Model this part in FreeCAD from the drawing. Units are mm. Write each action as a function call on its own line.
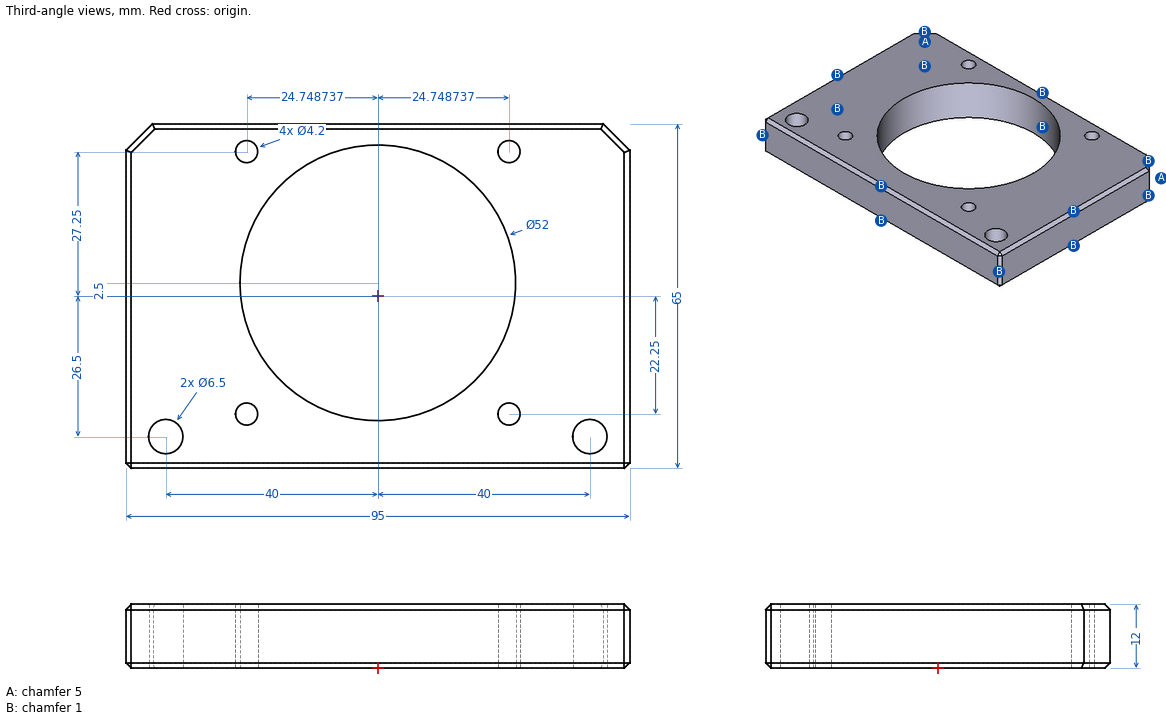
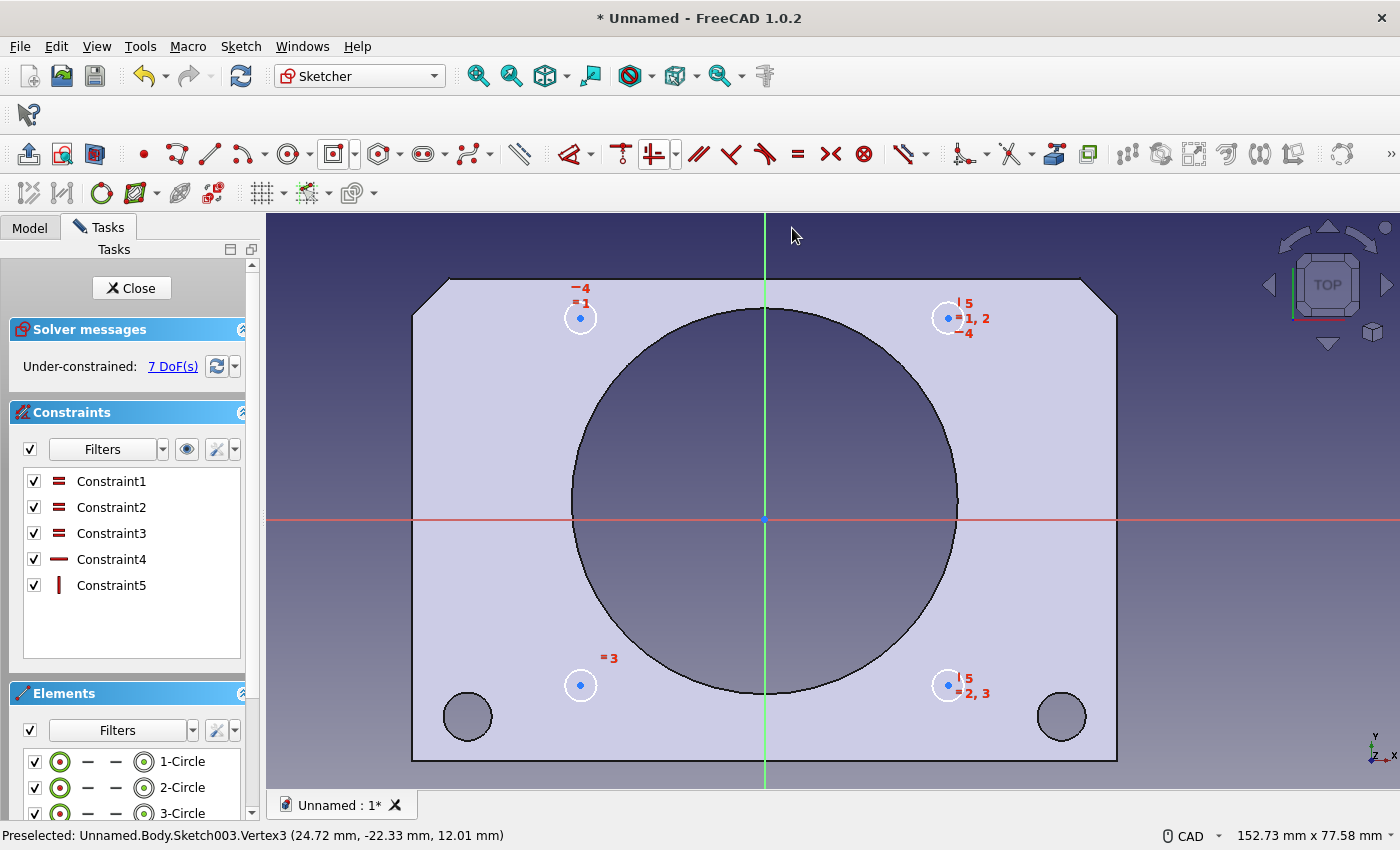
click(581, 318)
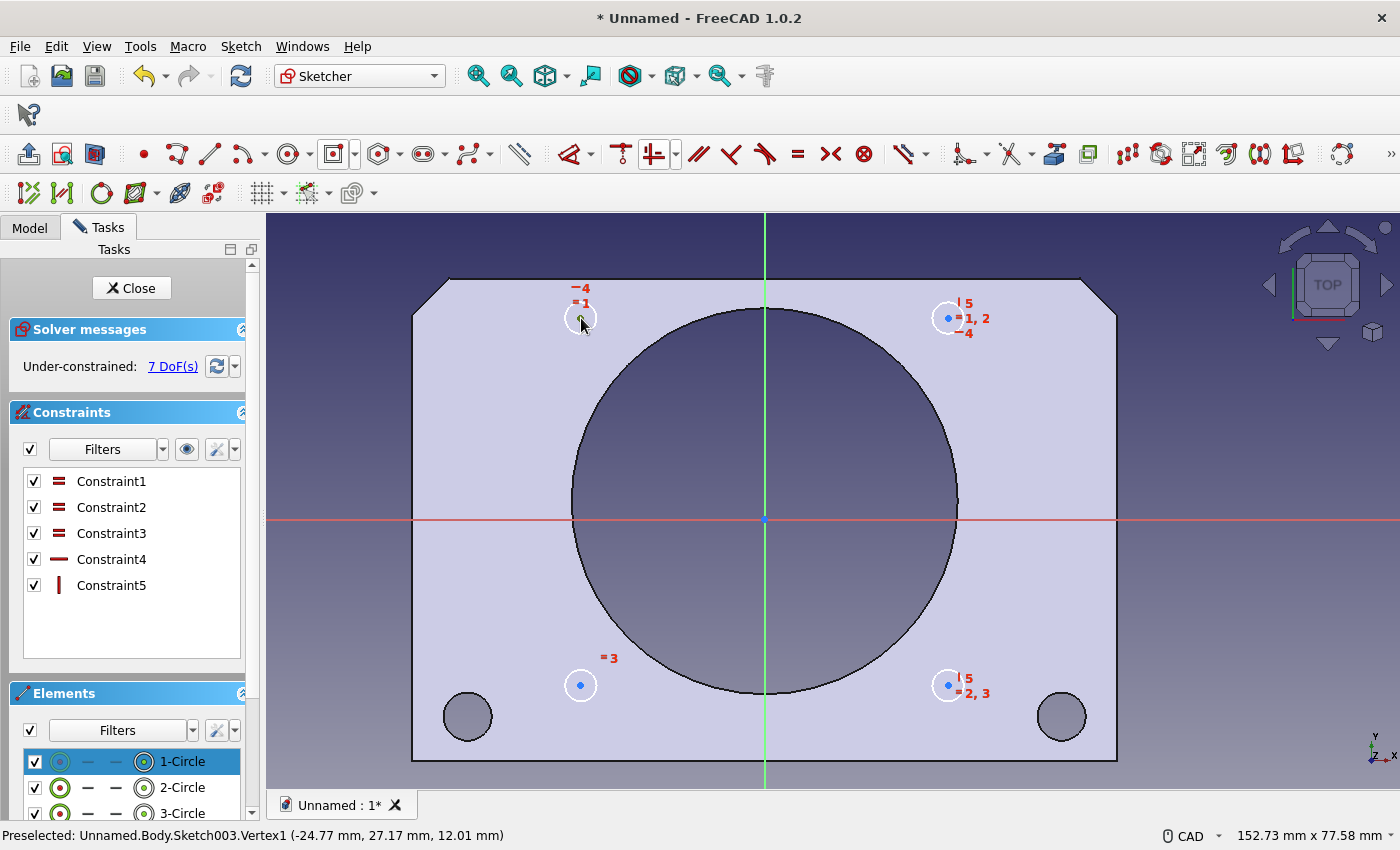
click(581, 686)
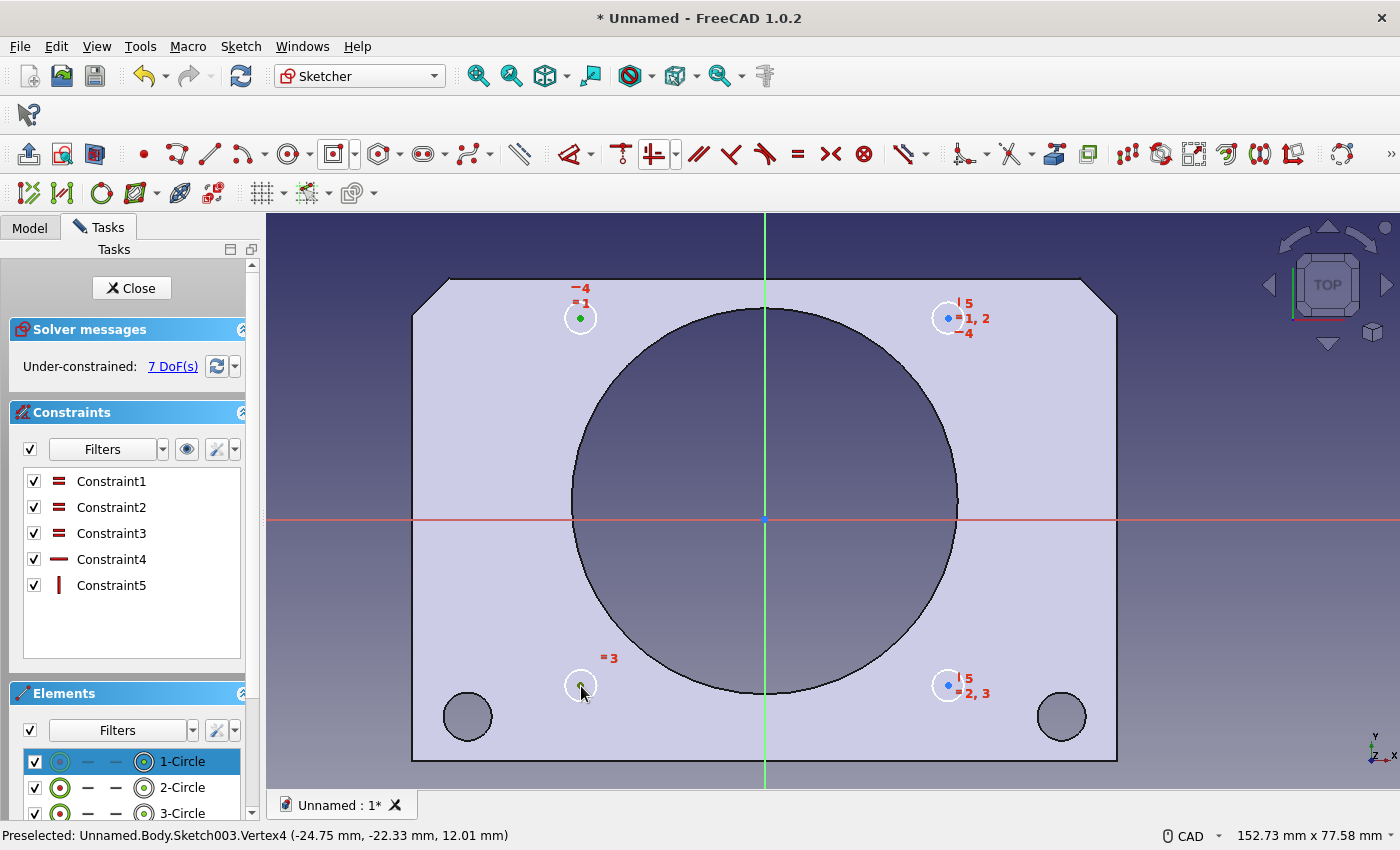
click(676, 154)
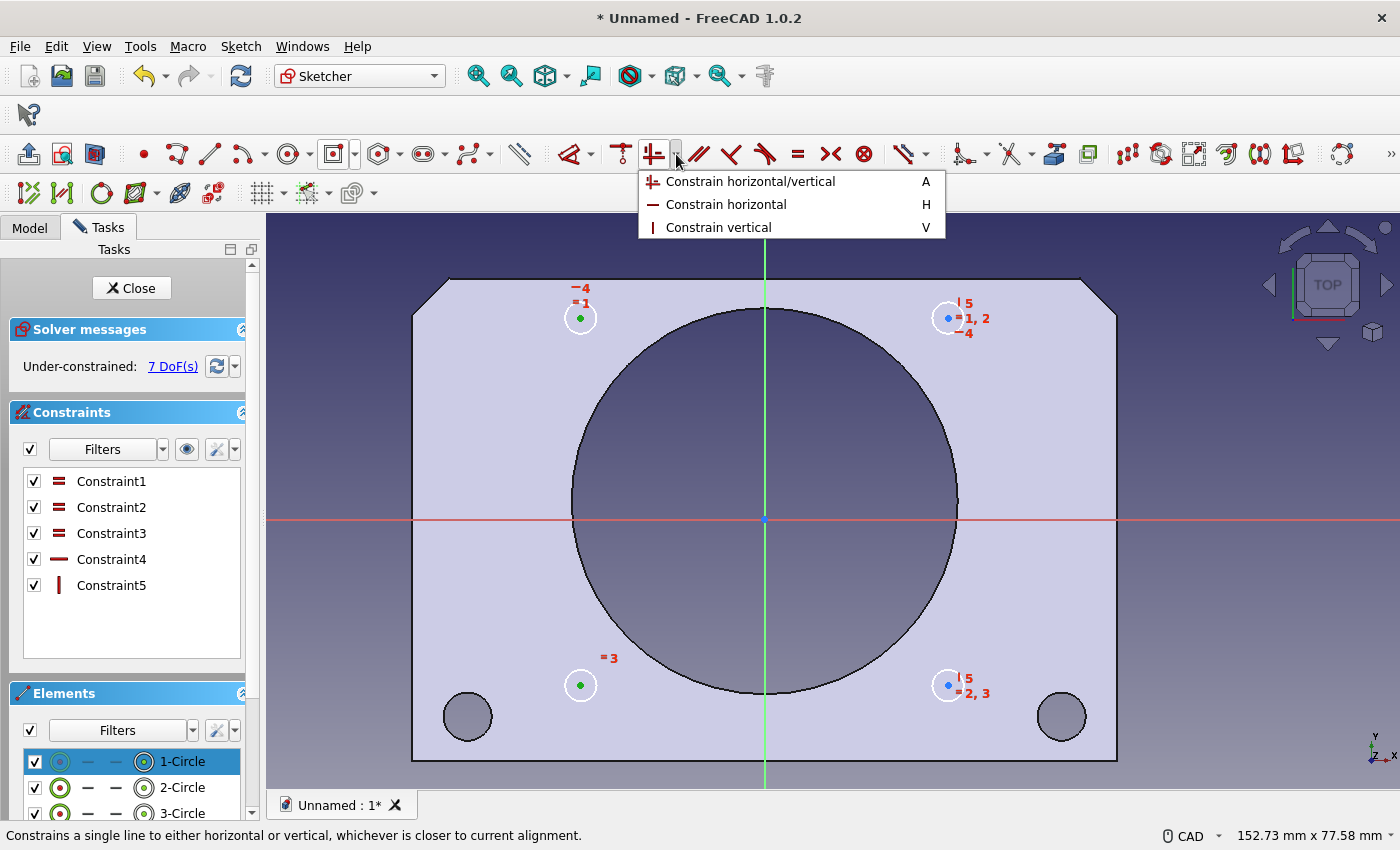
click(792, 228)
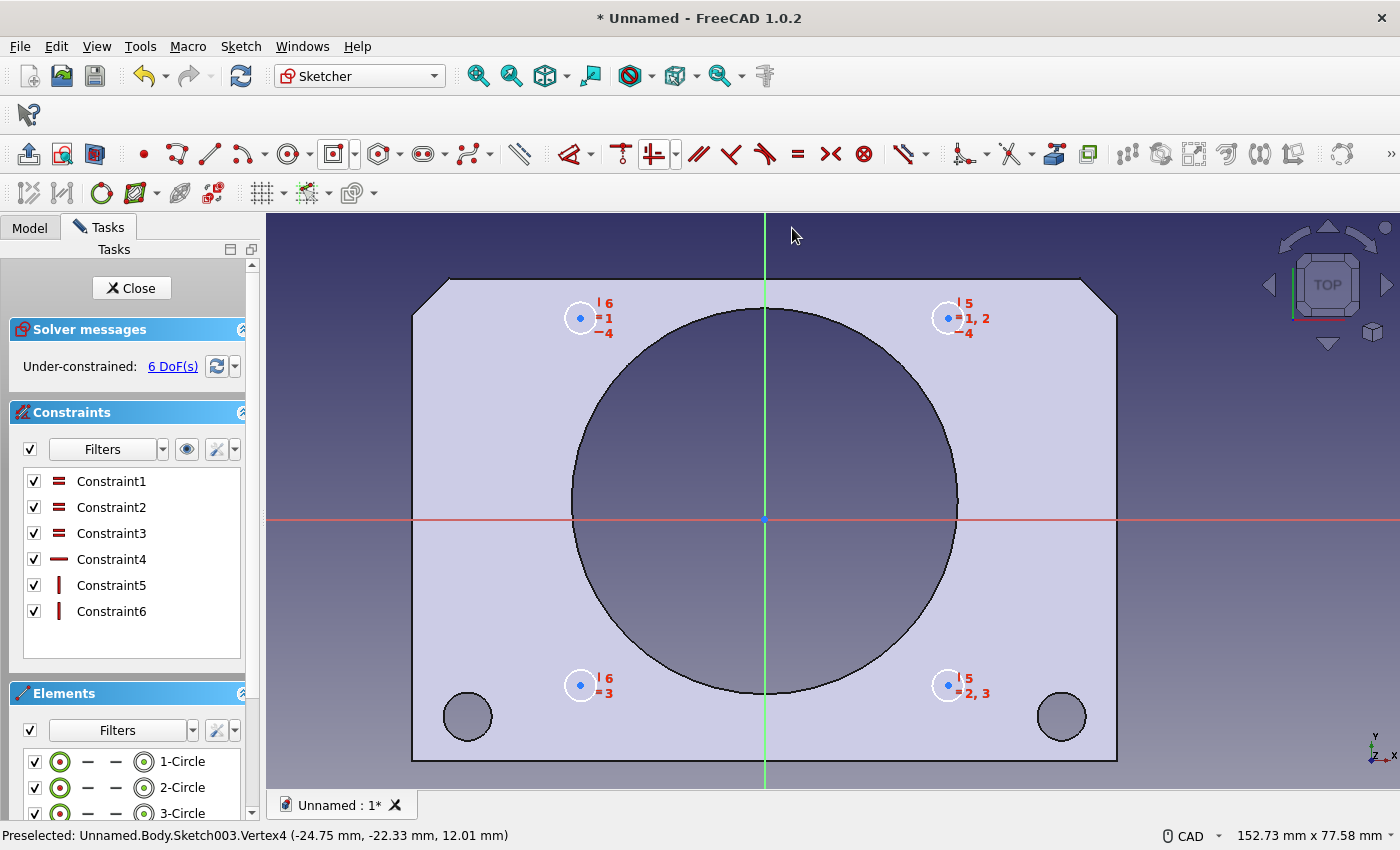
click(948, 686)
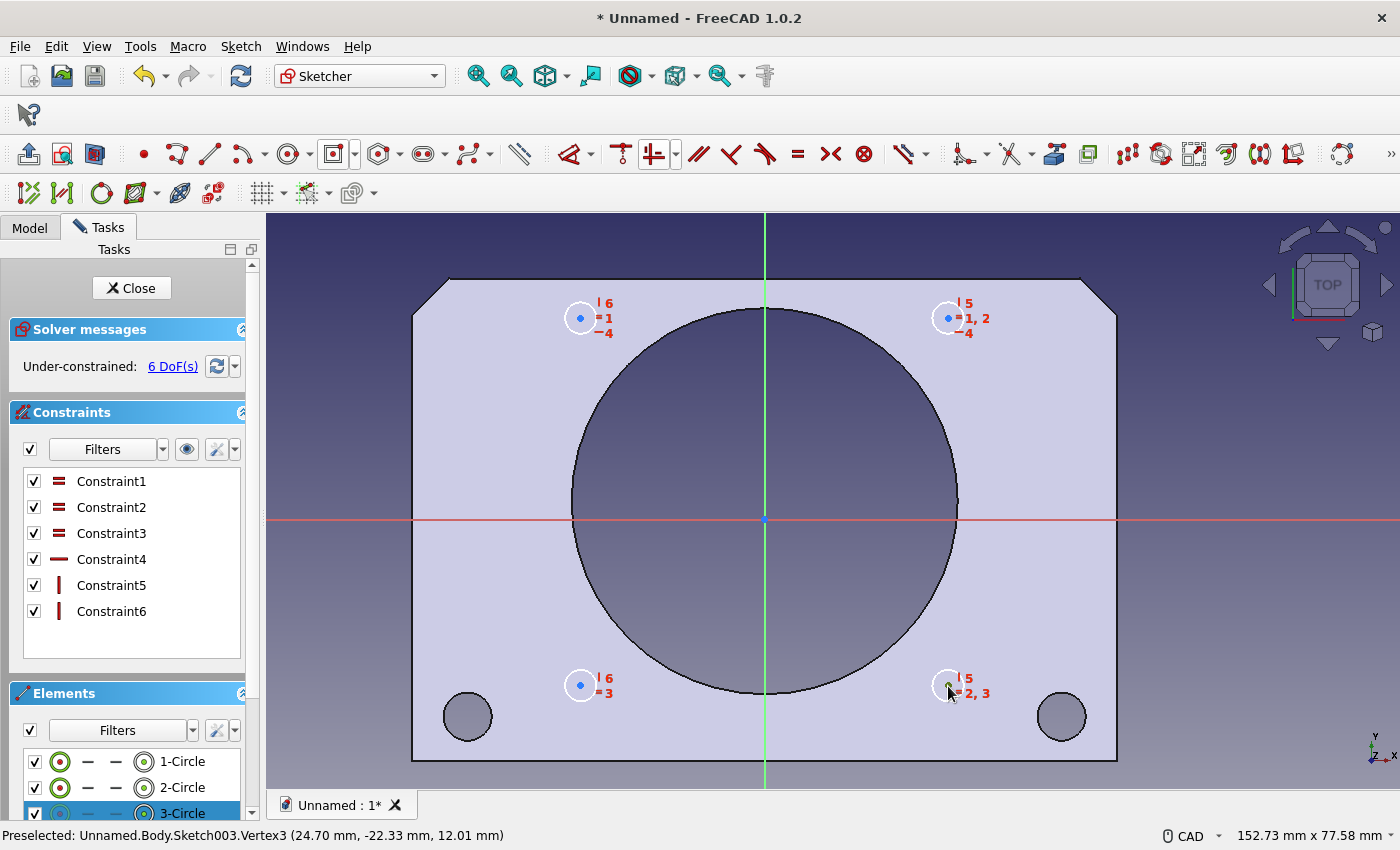
click(581, 686)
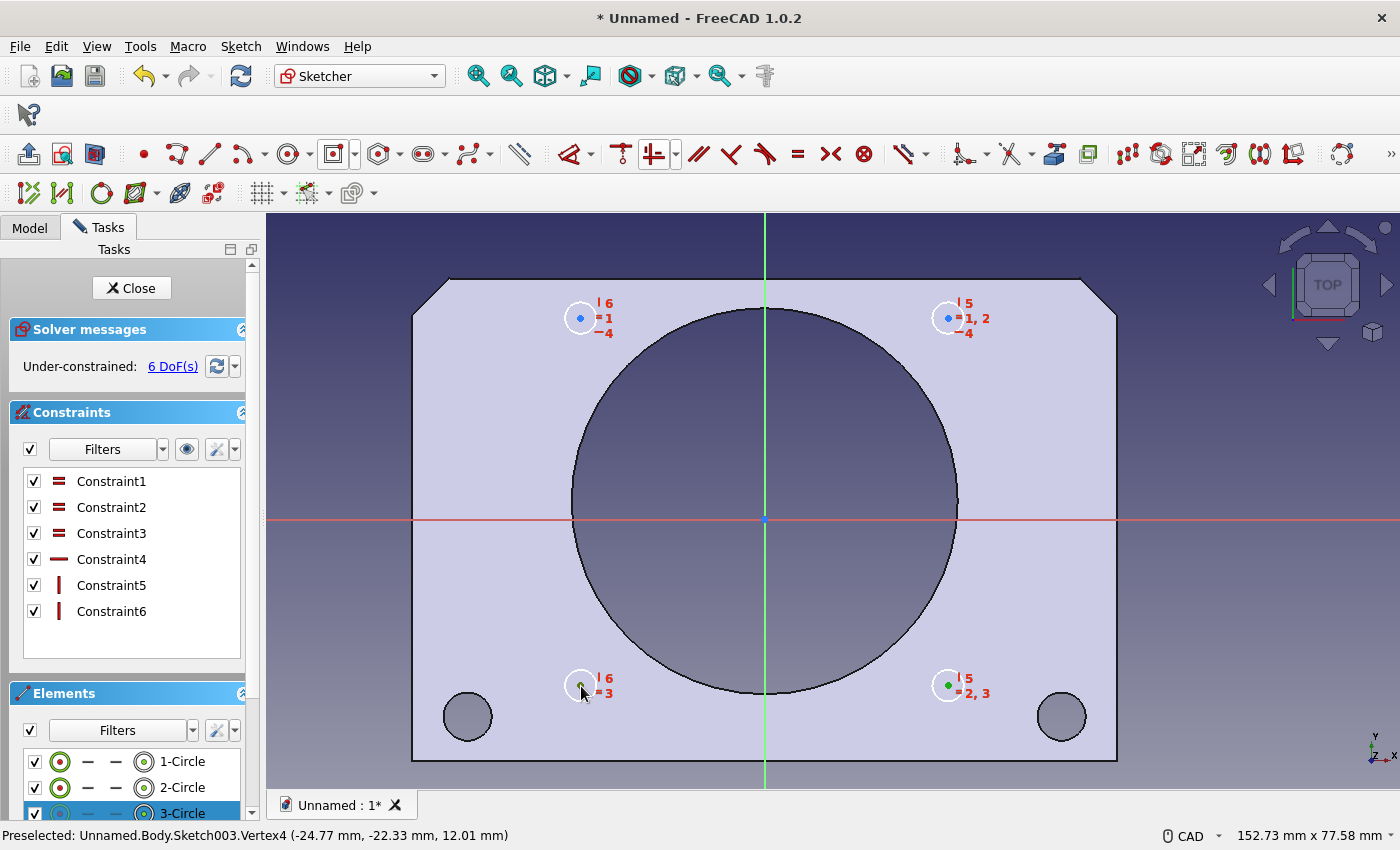
click(676, 154)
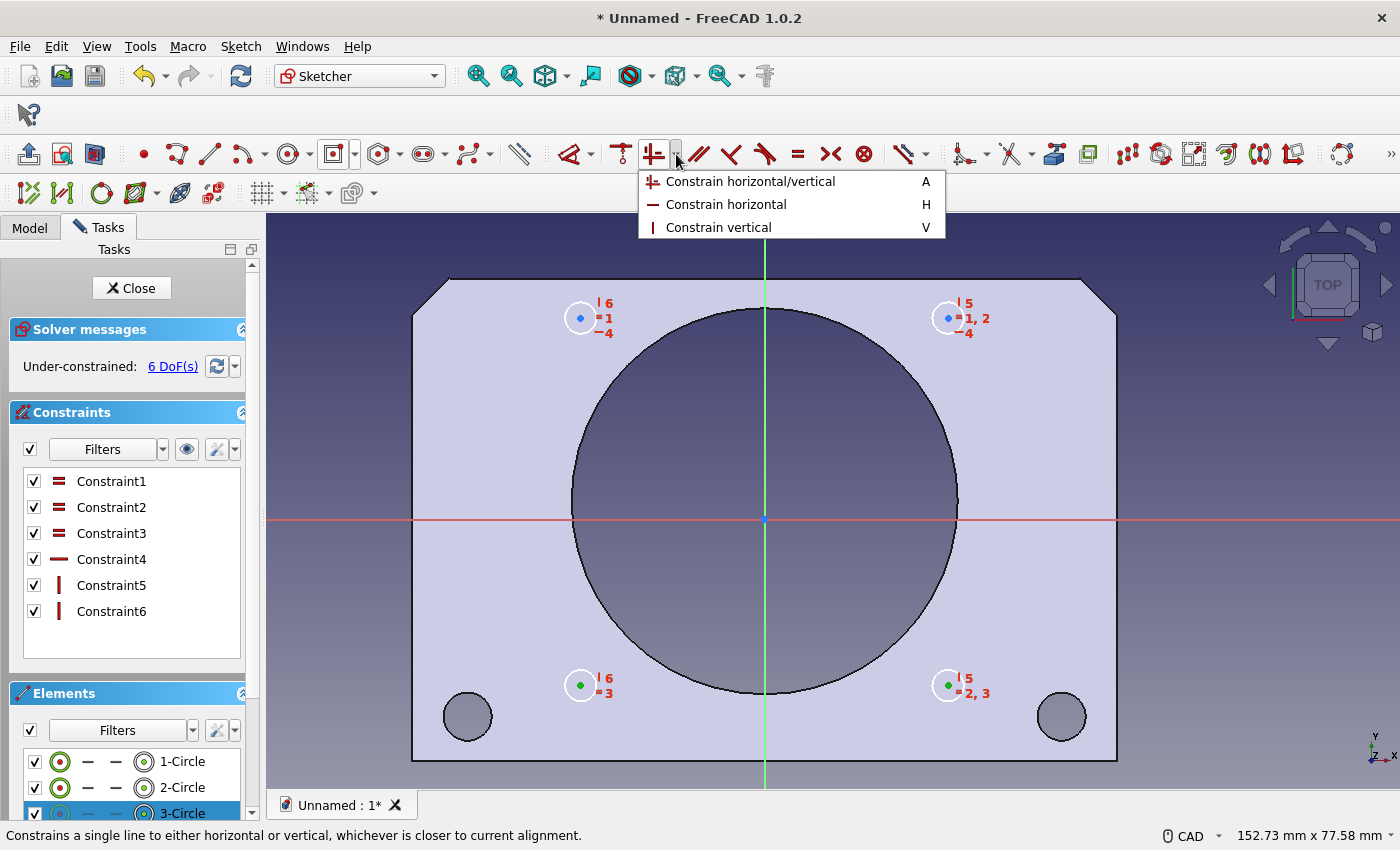
click(792, 204)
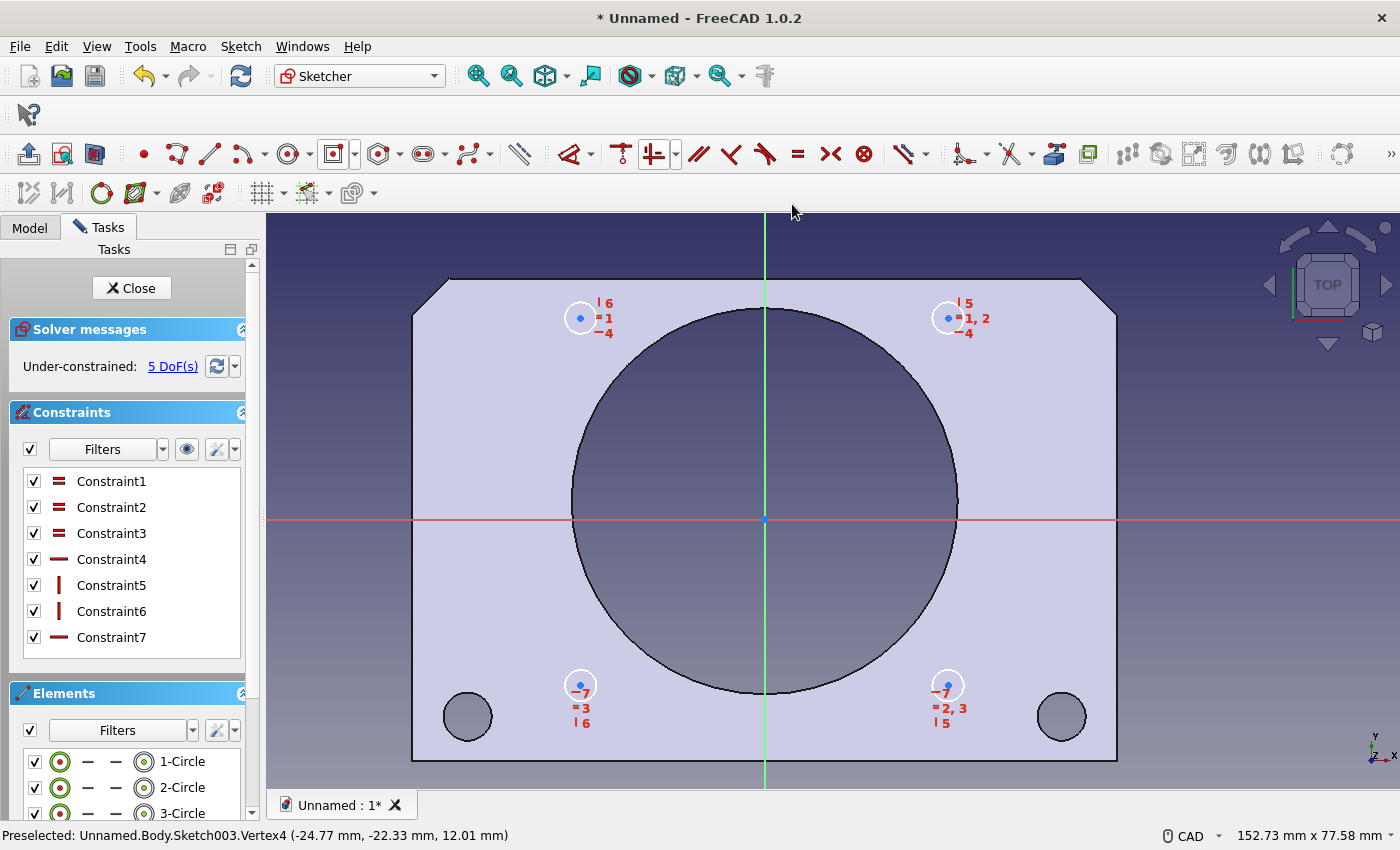
key(d)